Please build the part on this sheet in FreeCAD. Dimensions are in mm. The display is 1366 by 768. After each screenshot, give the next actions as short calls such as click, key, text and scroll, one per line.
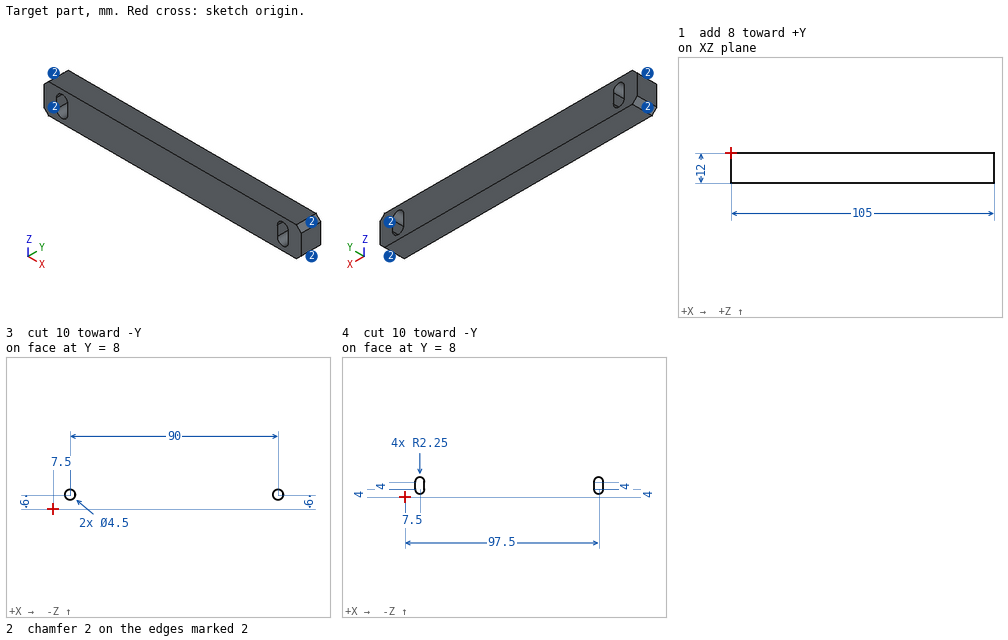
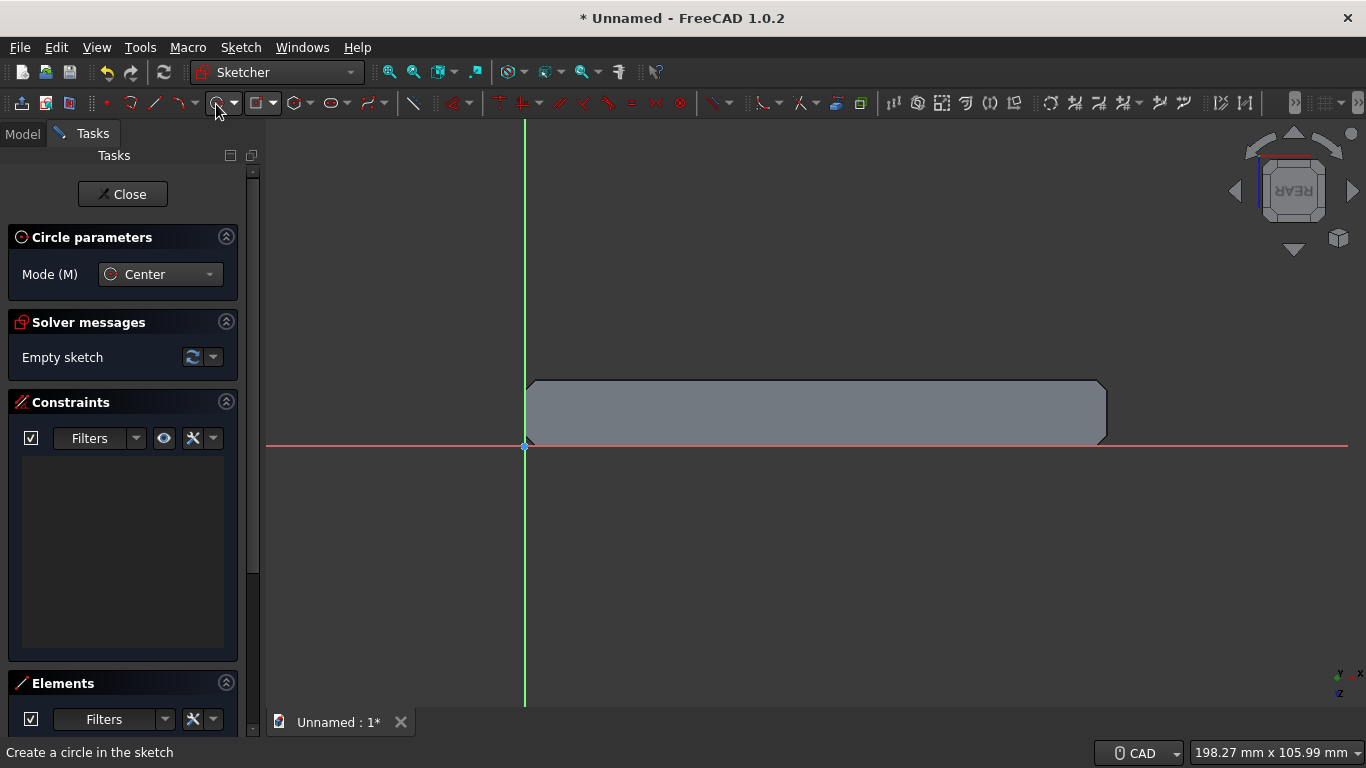
scroll(566, 413, up, 3)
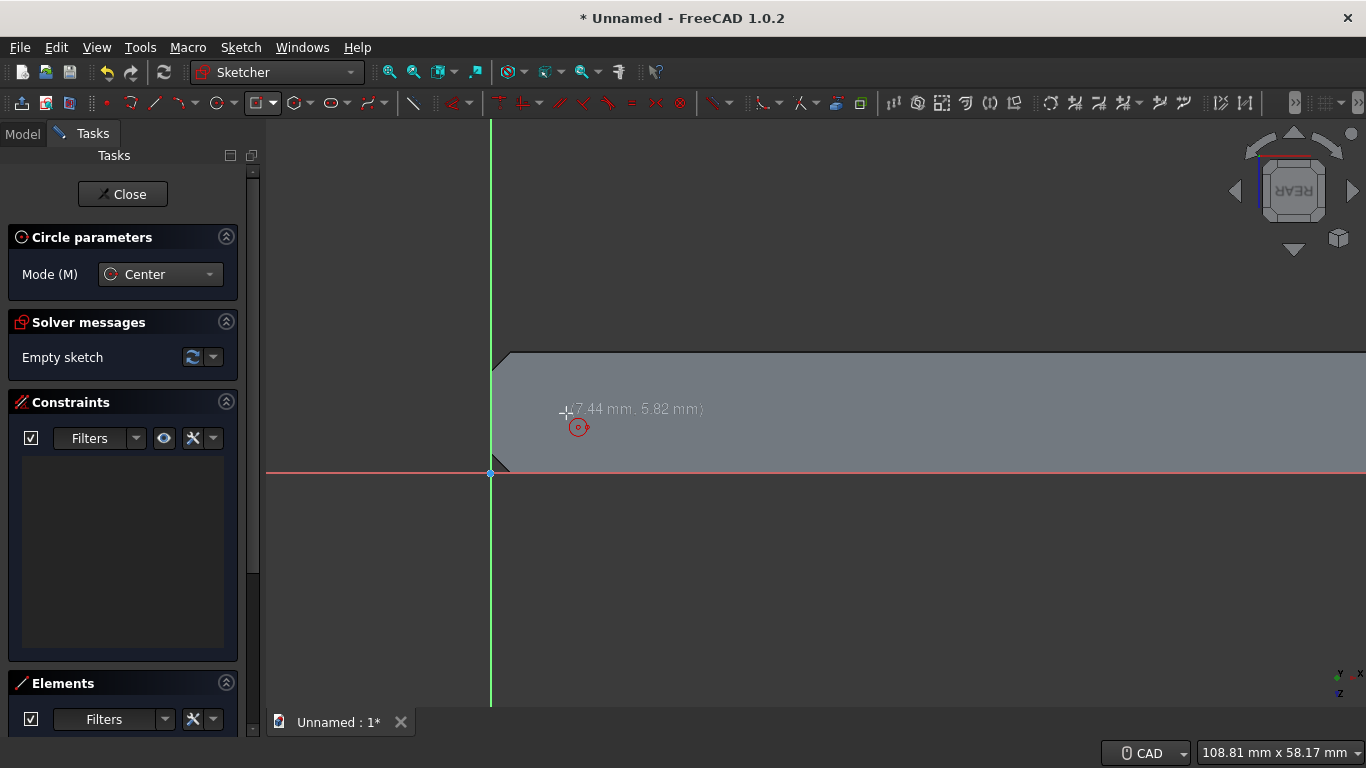
click(566, 413)
click(582, 397)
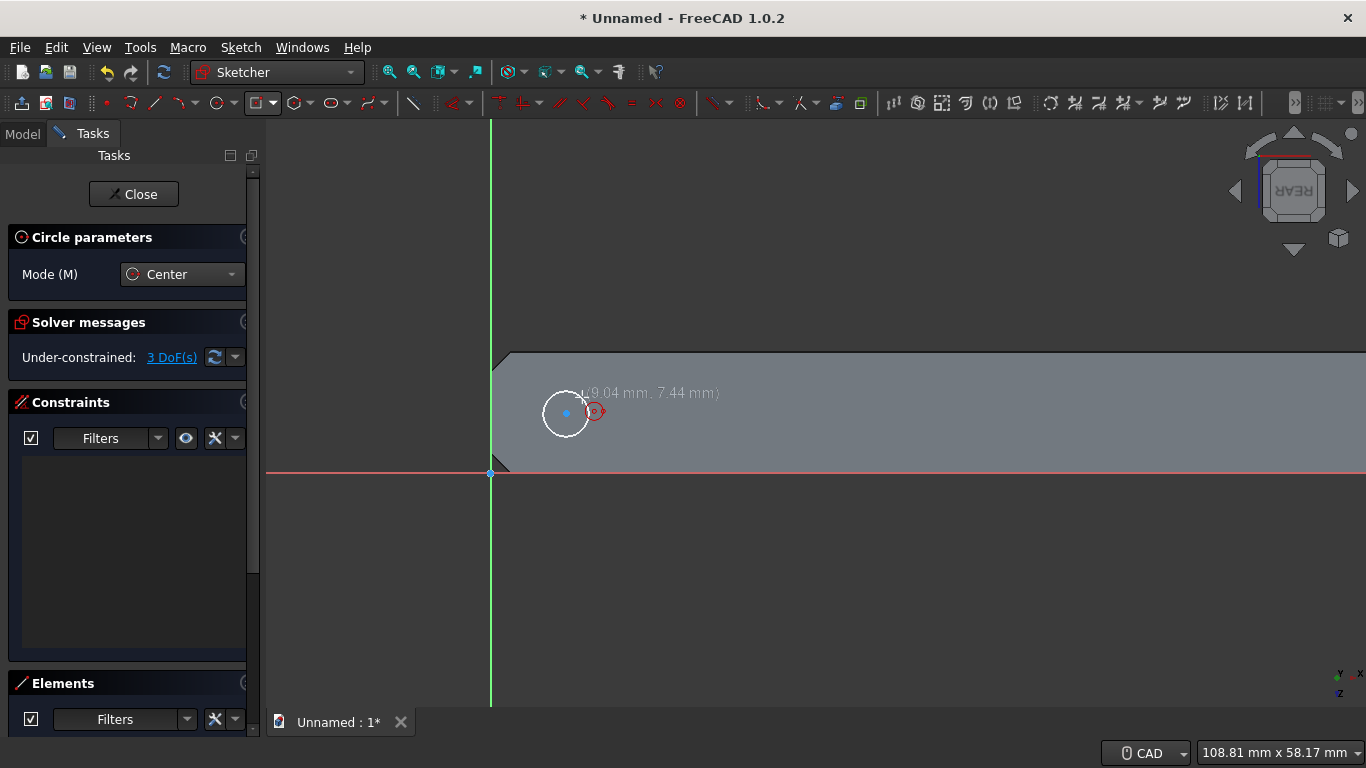
scroll(294, 375, down, 2)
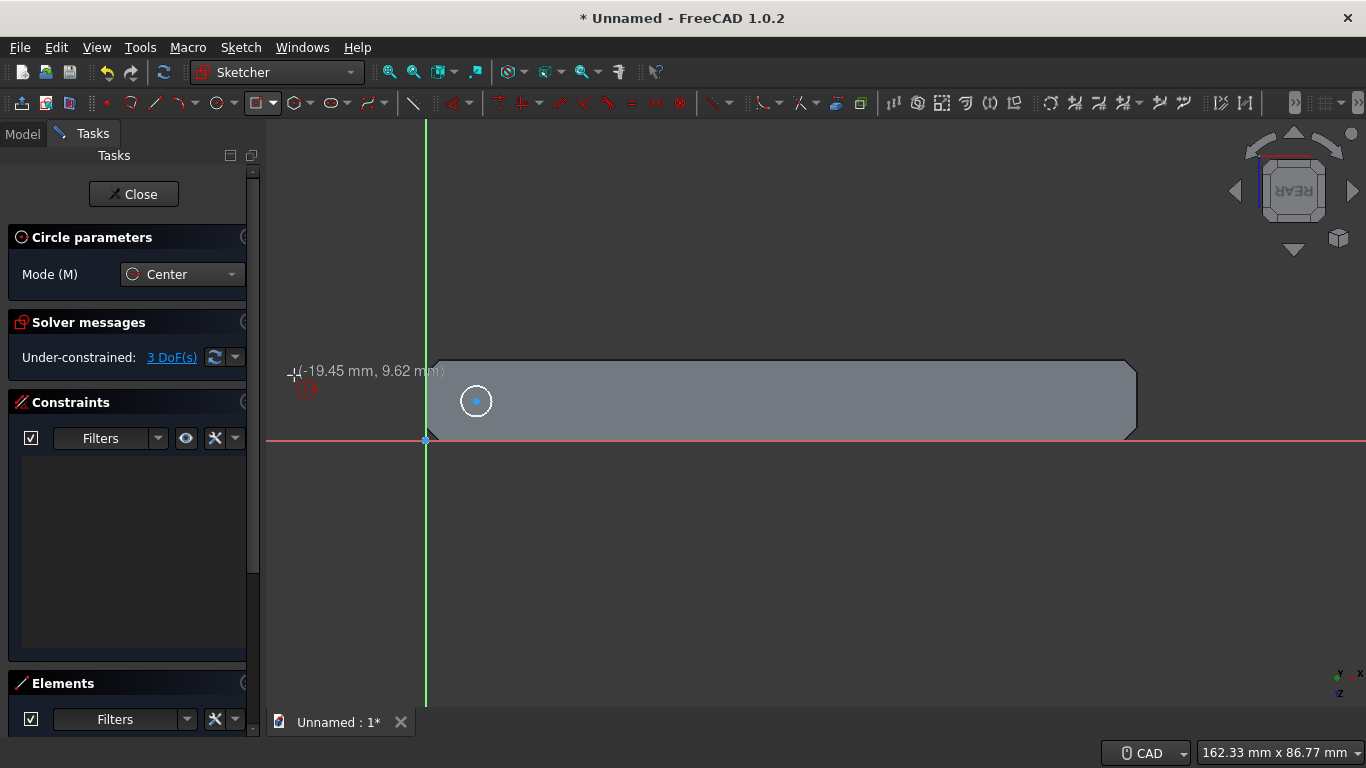
scroll(1086, 400, up, 2)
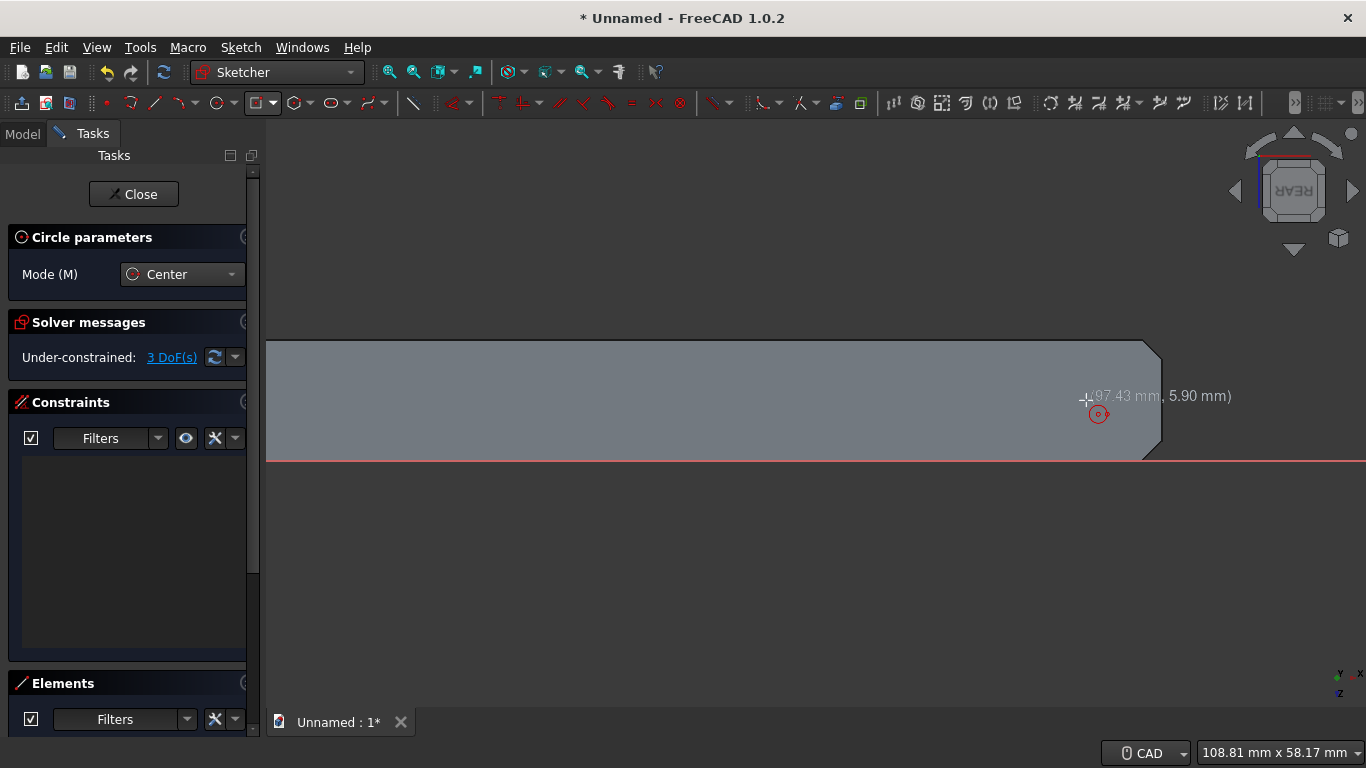
click(1086, 400)
click(1102, 384)
key(Escape)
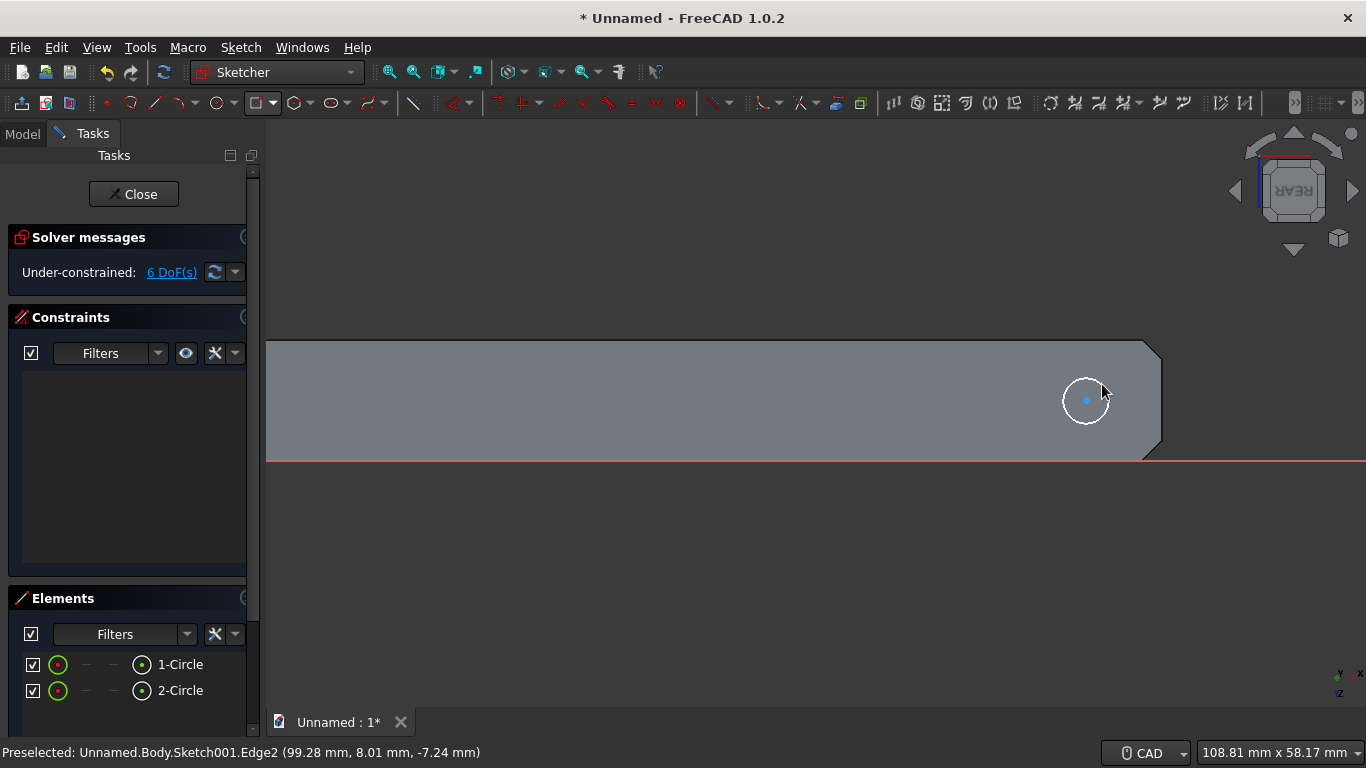
scroll(1037, 400, down, 2)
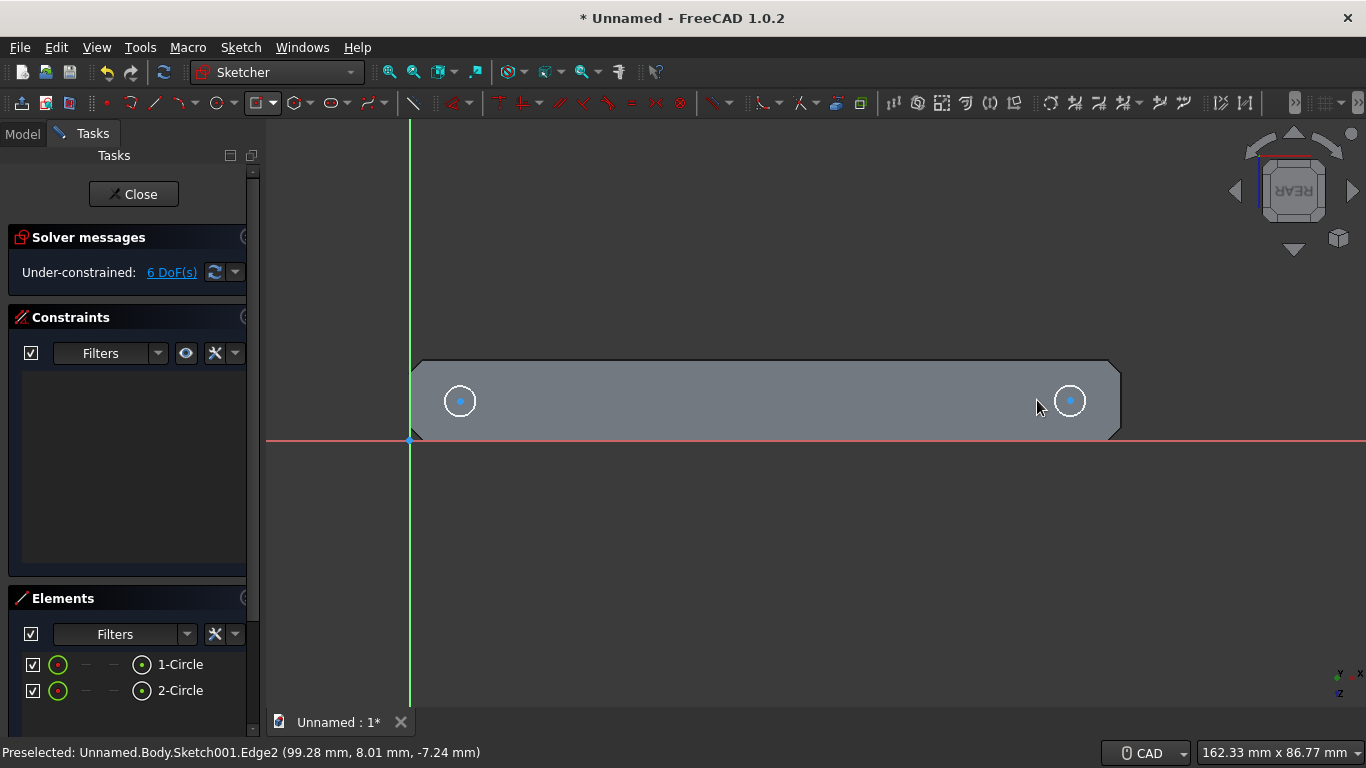
click(471, 391)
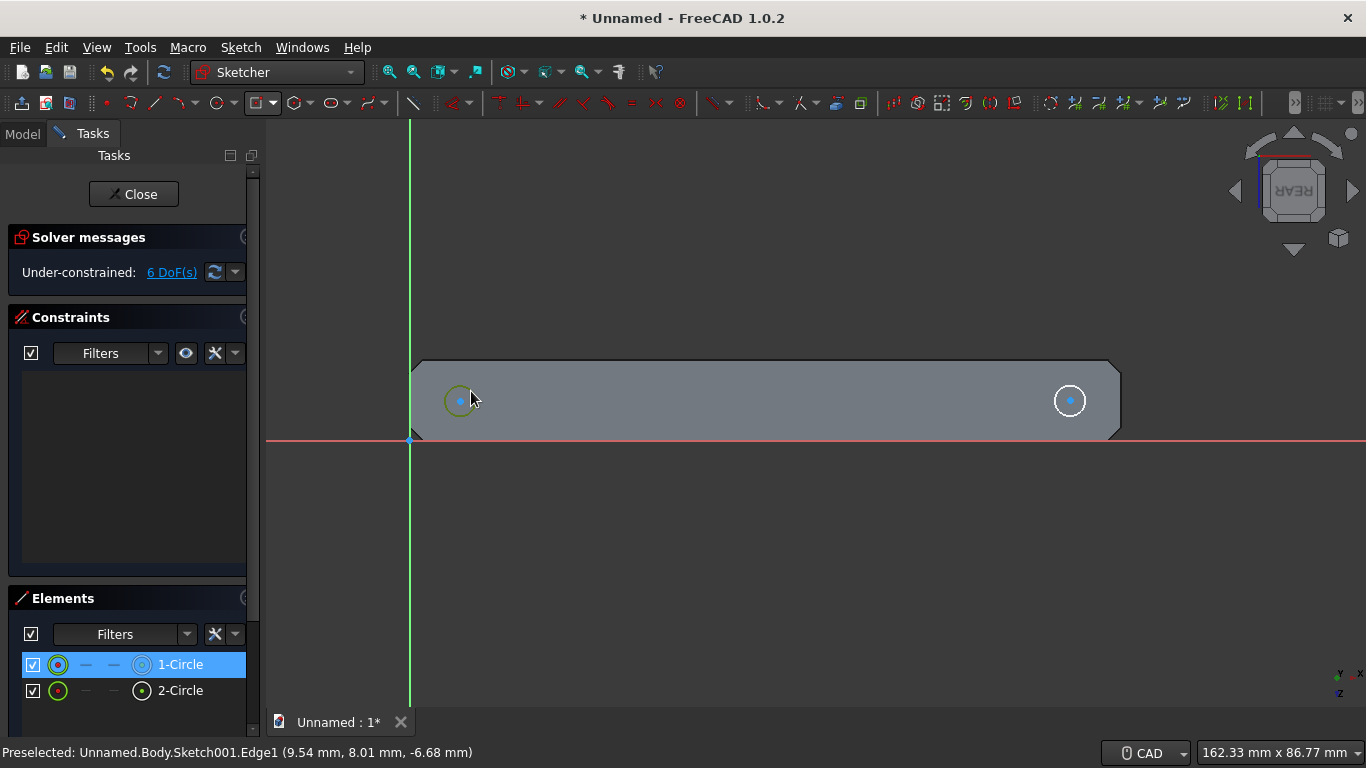
click(1081, 390)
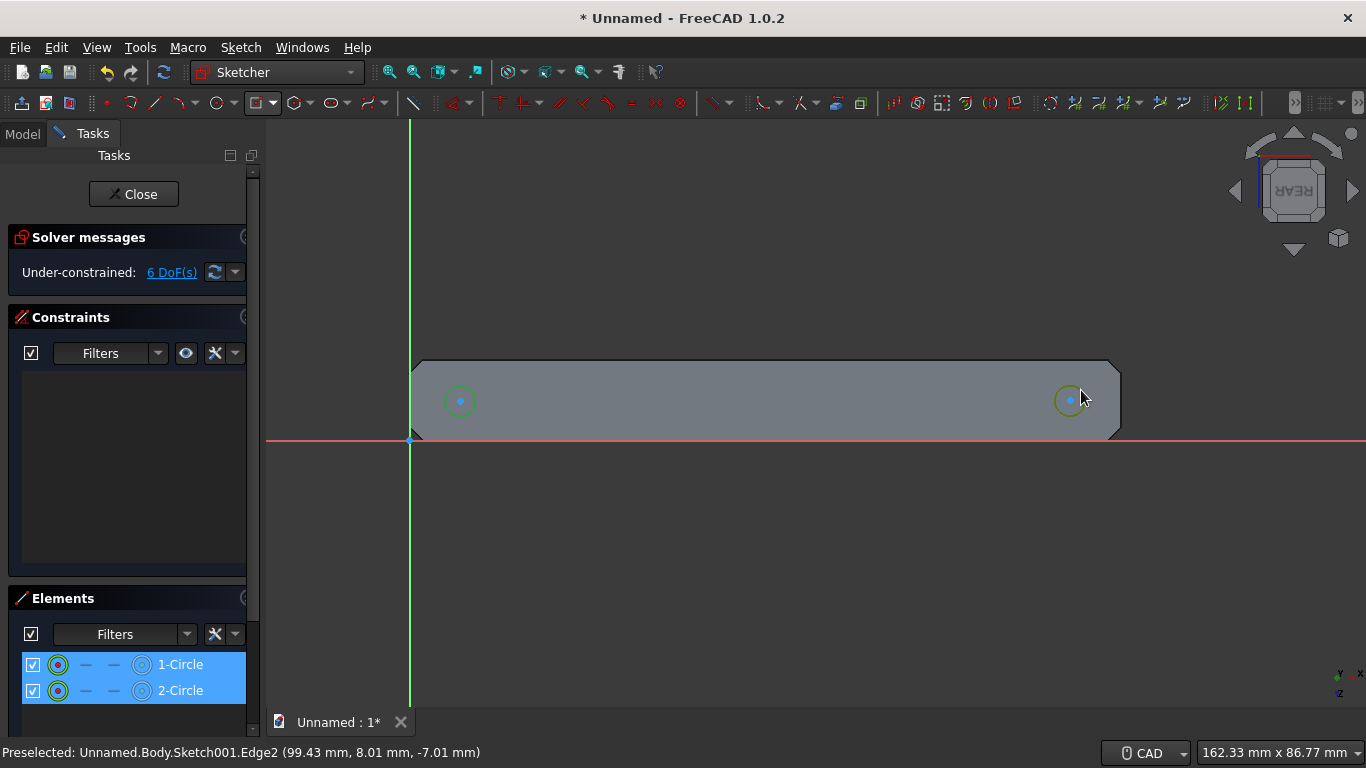
click(632, 104)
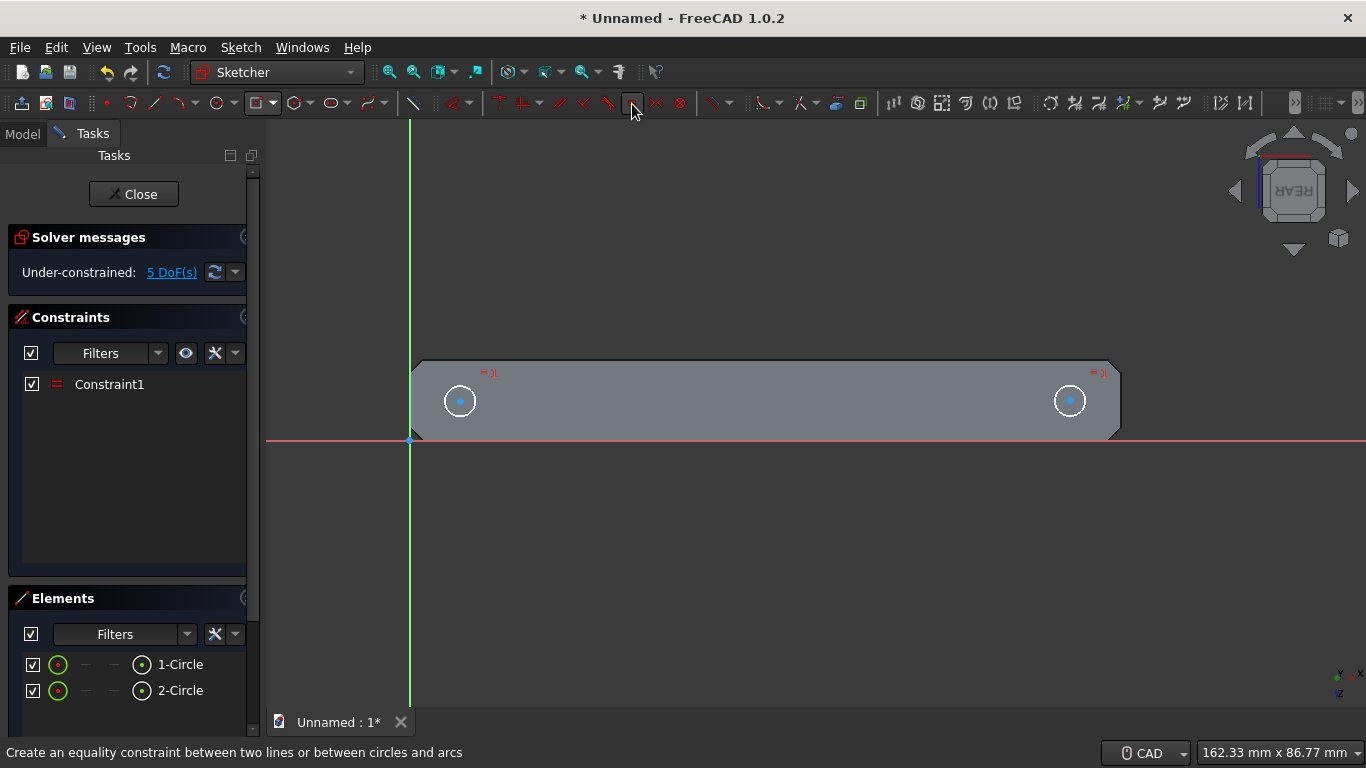
click(452, 104)